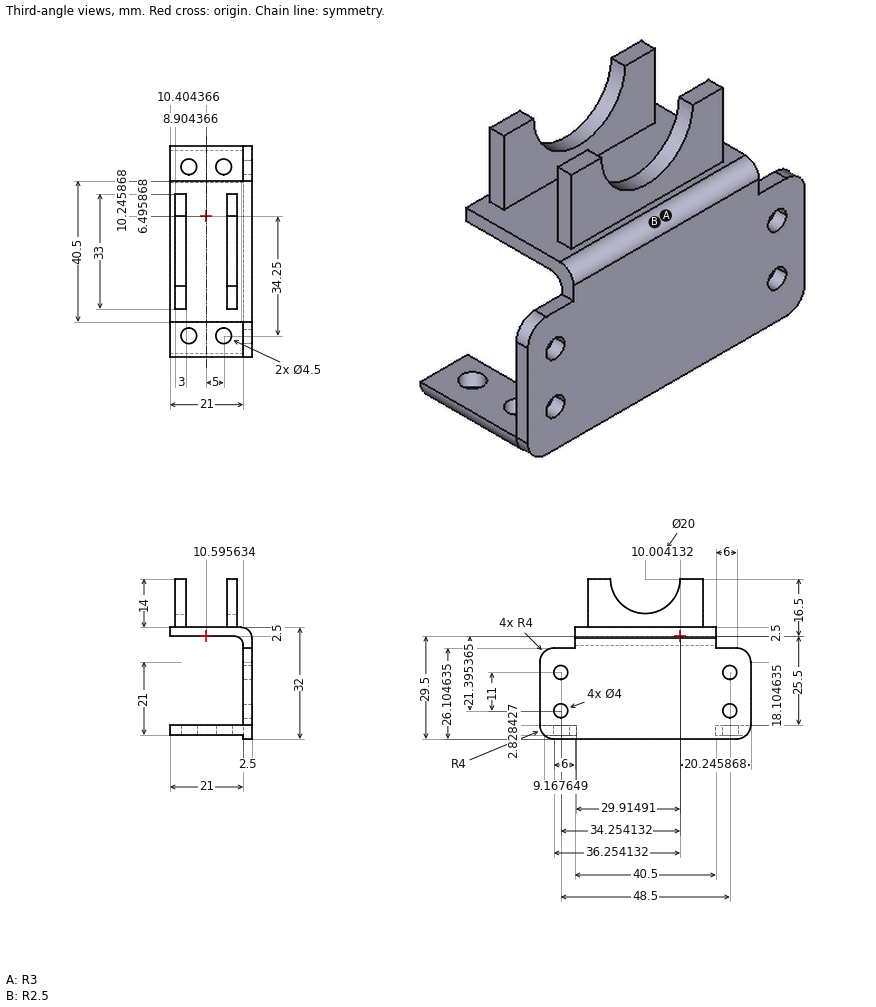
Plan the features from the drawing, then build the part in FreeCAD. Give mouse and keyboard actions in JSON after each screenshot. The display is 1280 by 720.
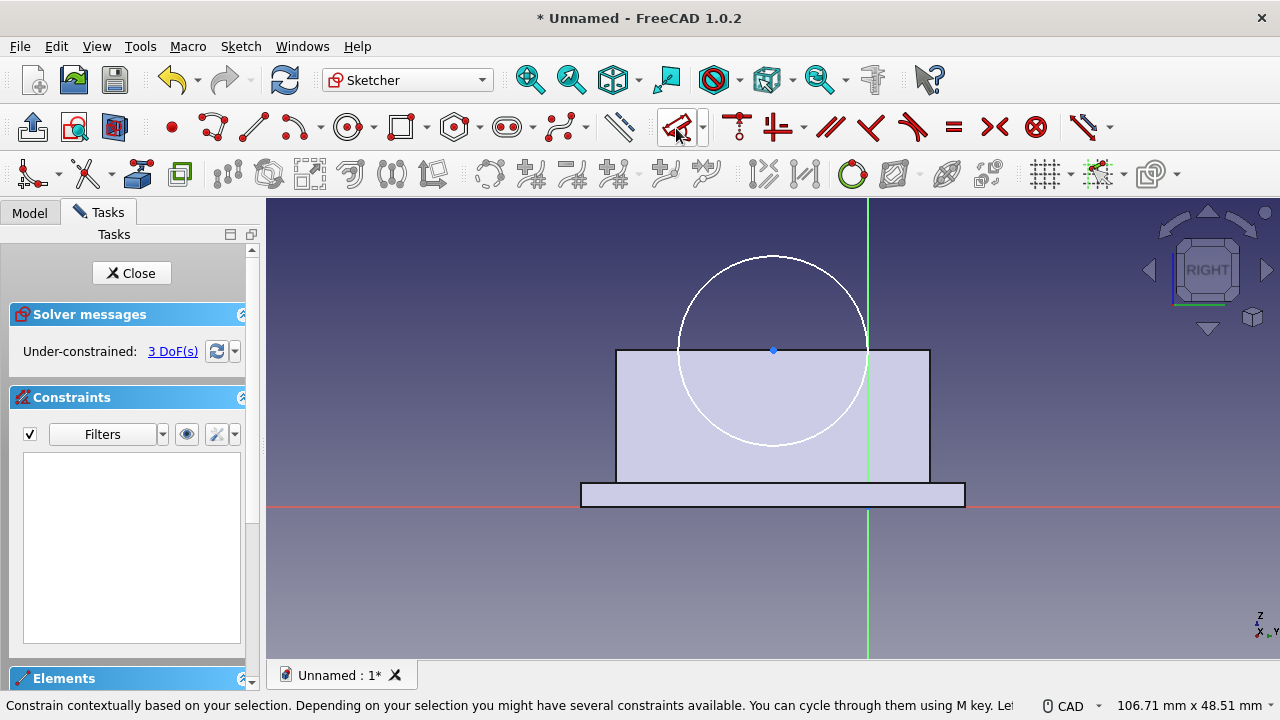
{"action": "left_click", "coordinate": [840, 284]}
{"action": "left_click", "coordinate": [895, 315]}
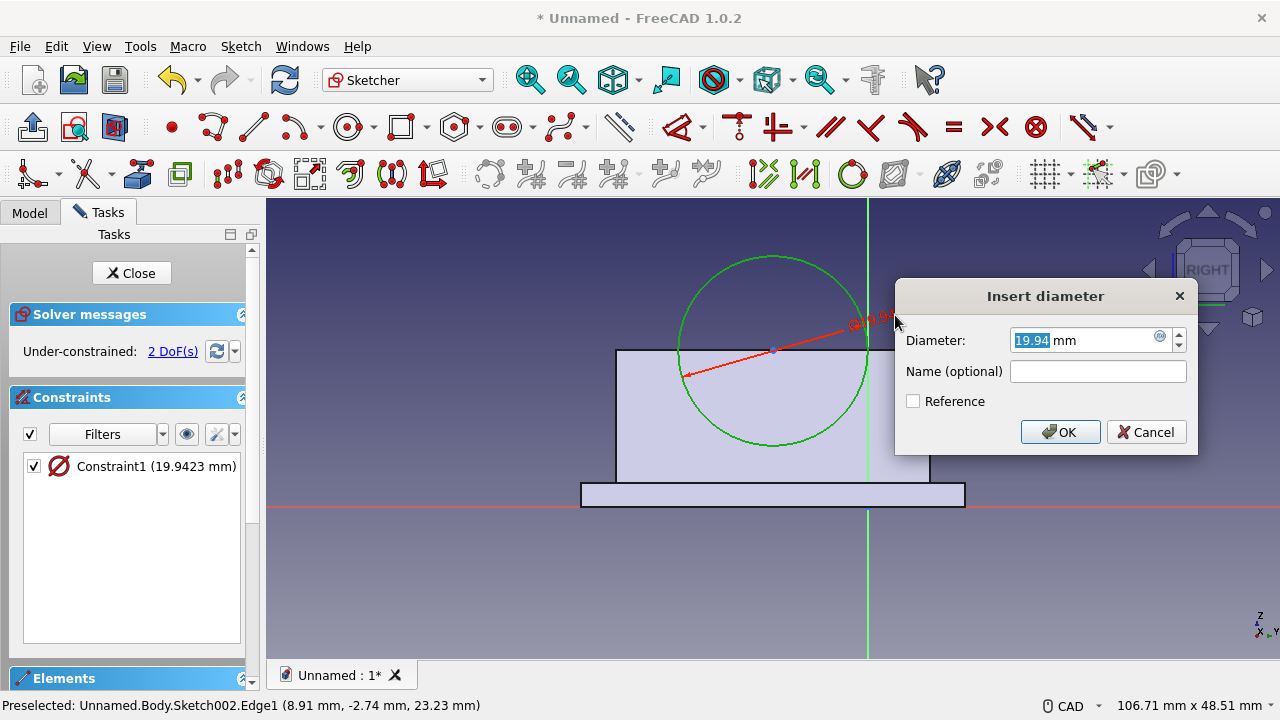
{"action": "type", "text": "20"}
{"action": "key", "text": "Return"}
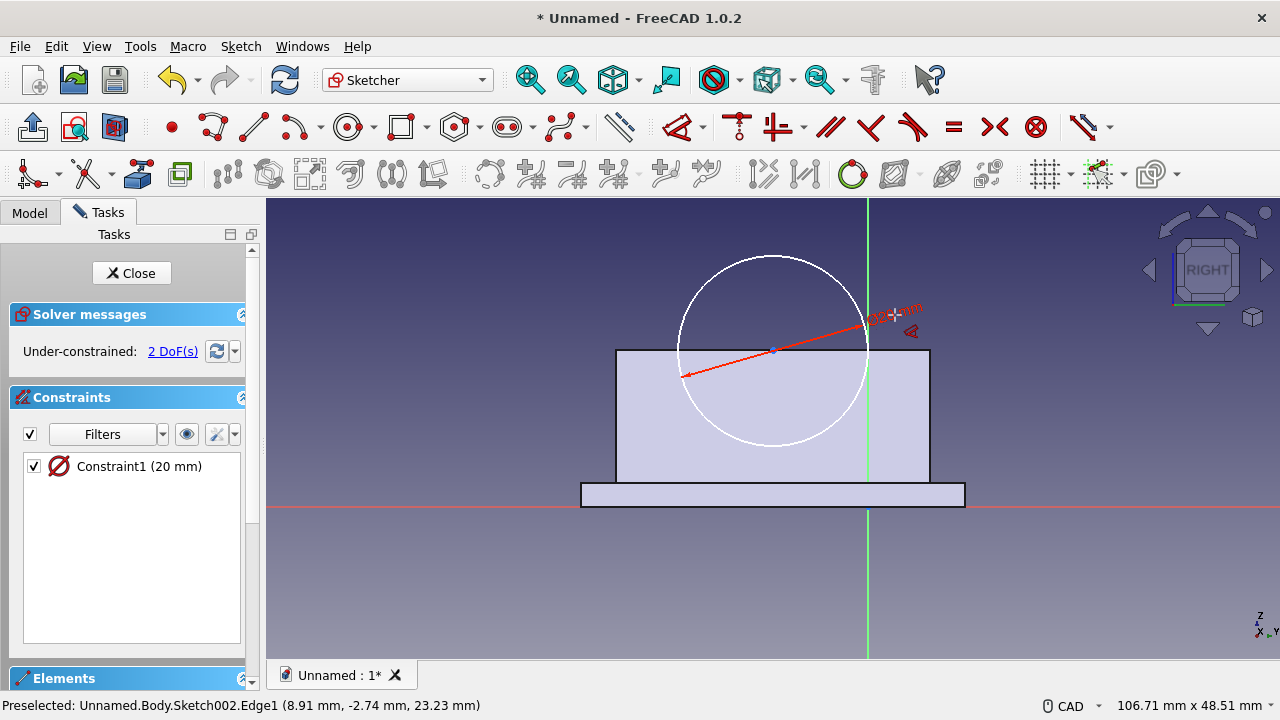
{"action": "left_click", "coordinate": [773, 351]}
{"action": "left_click", "coordinate": [902, 429]}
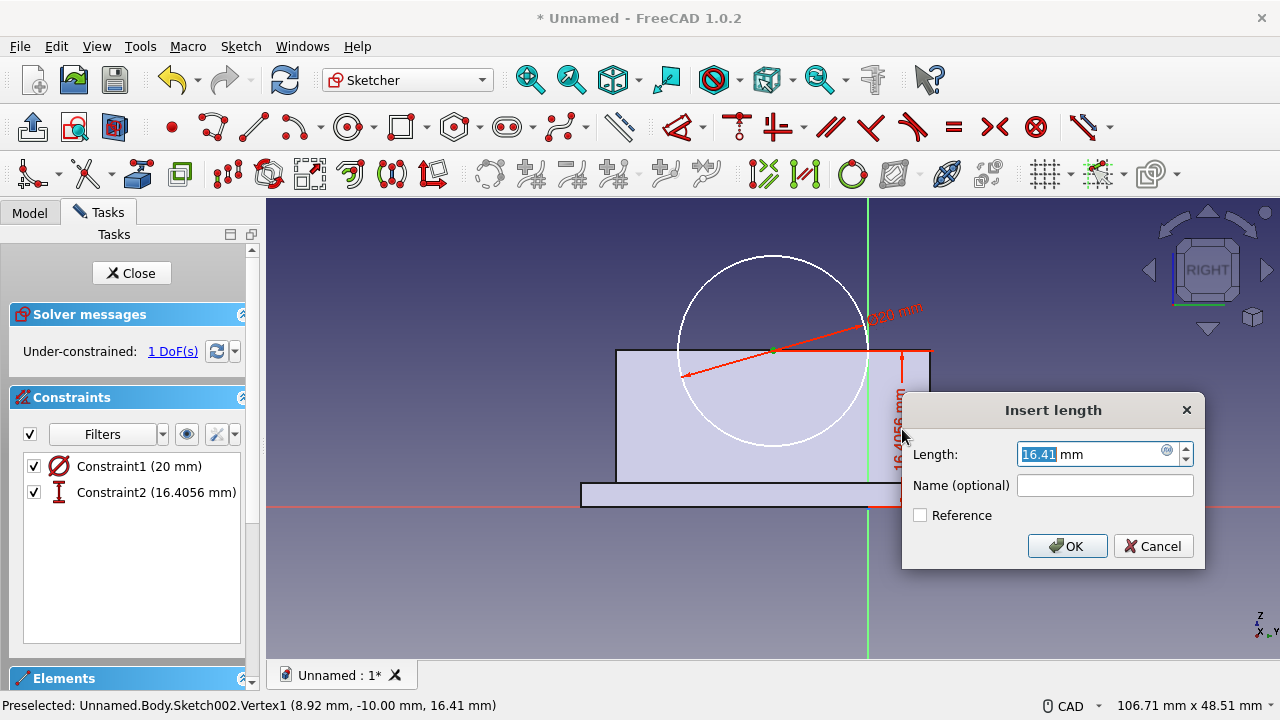
{"action": "type", "text": "16.5"}
{"action": "key", "text": "Return"}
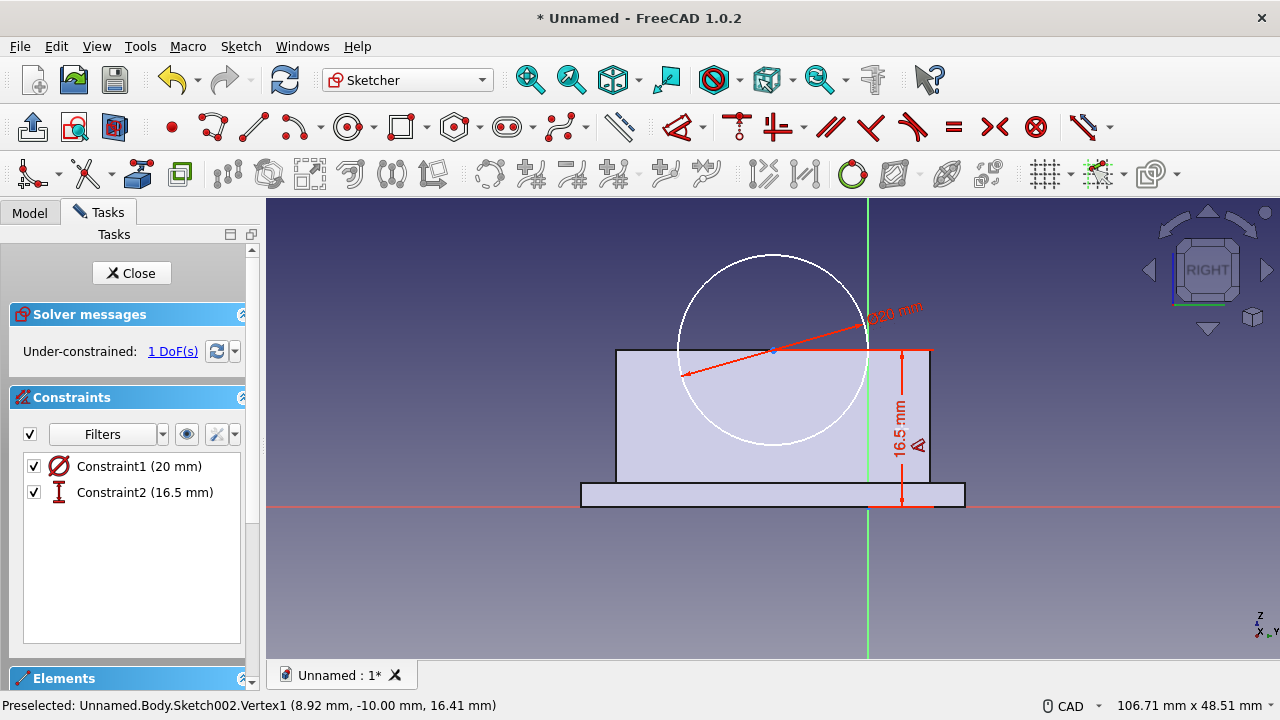
{"action": "left_click", "coordinate": [773, 350]}
{"action": "left_click", "coordinate": [821, 541]}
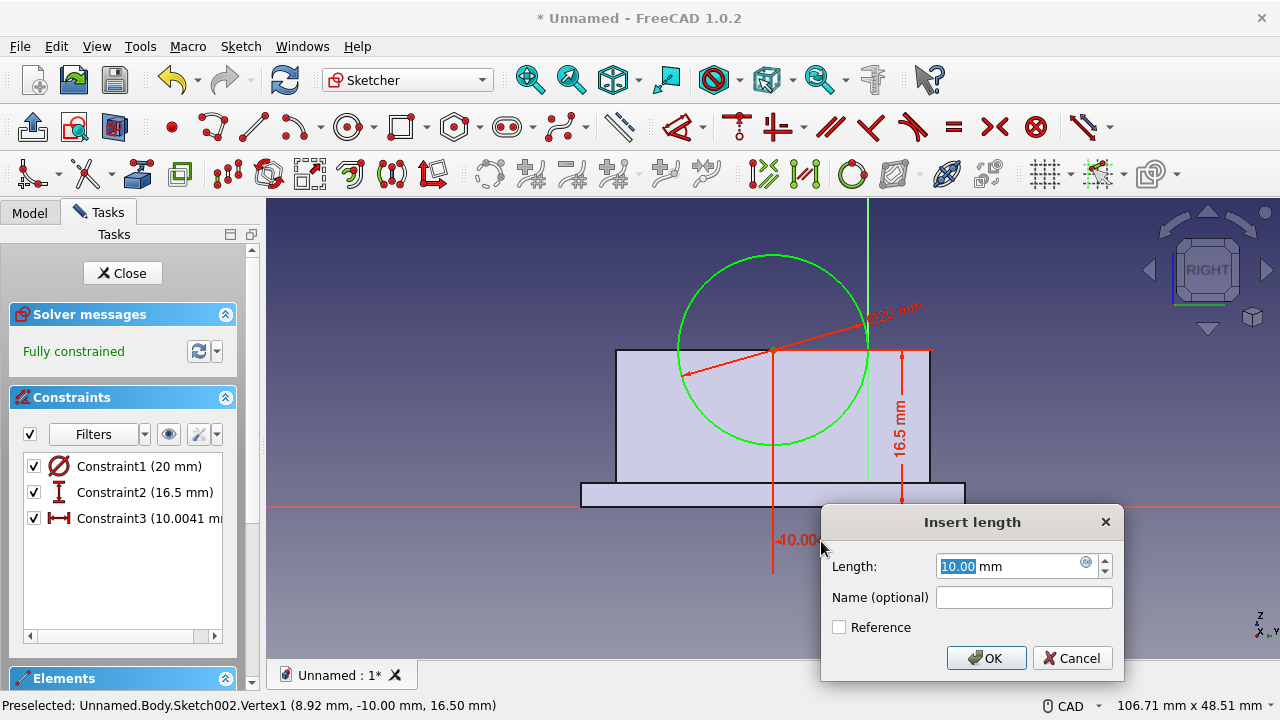
{"action": "type", "text": "10.004132"}
{"action": "key", "text": "Return"}
{"action": "key", "text": "Escape"}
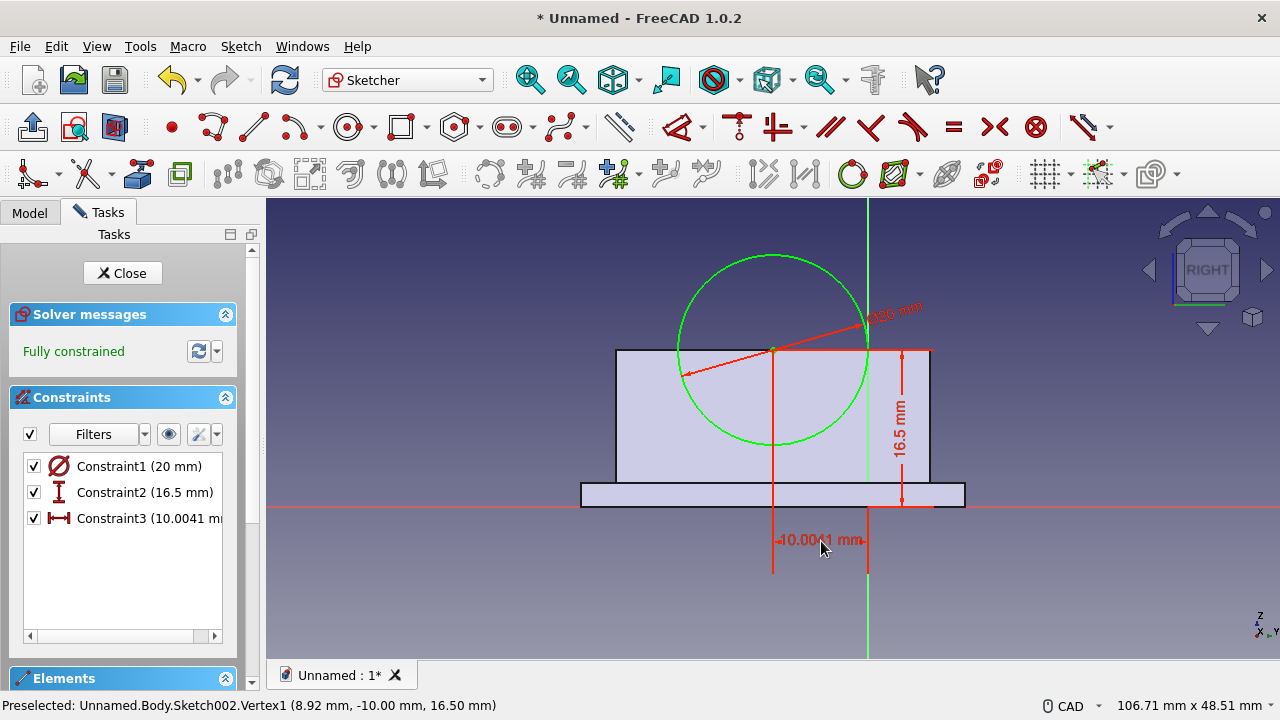
{"action": "left_click", "coordinate": [123, 273]}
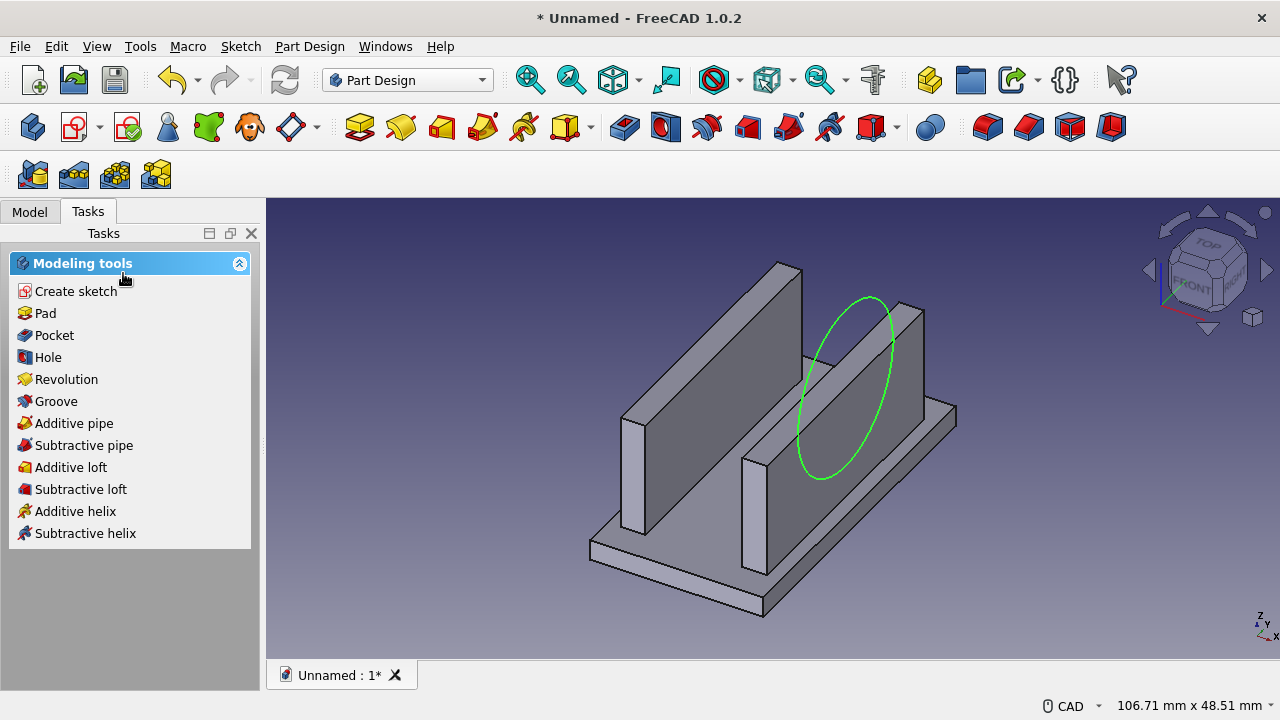
{"action": "left_click", "coordinate": [625, 128]}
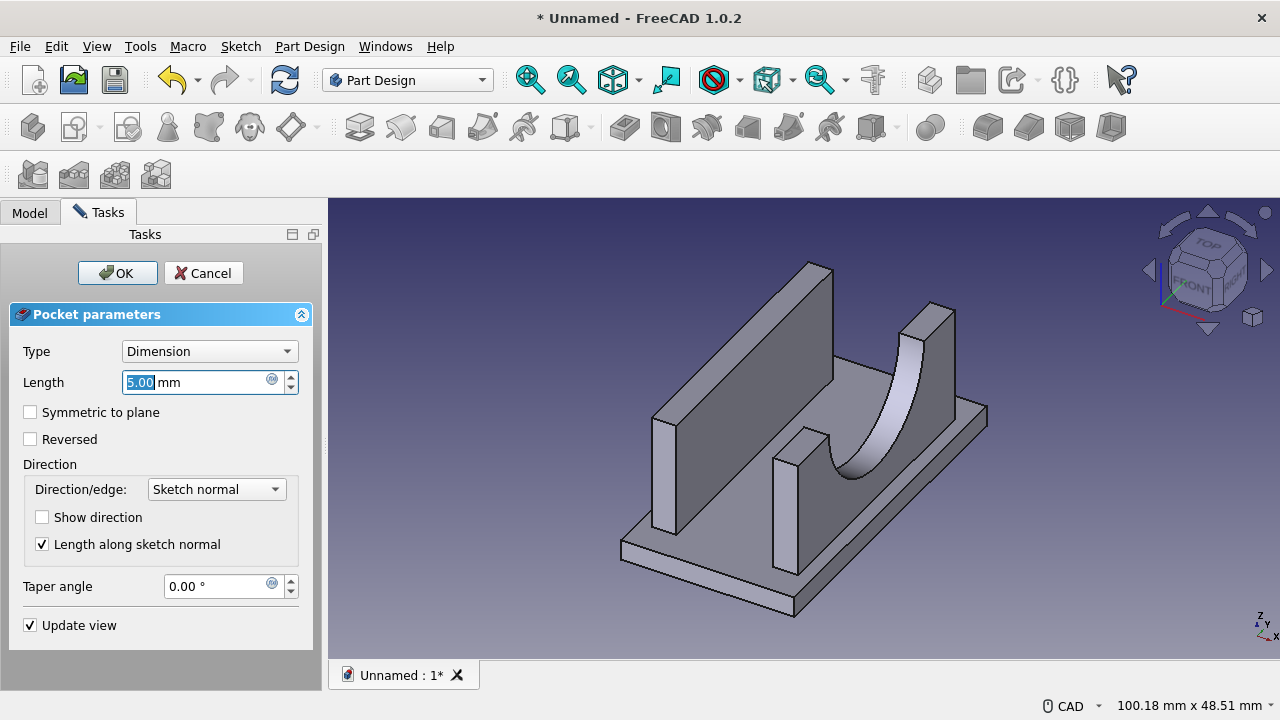
{"action": "left_click", "coordinate": [210, 352]}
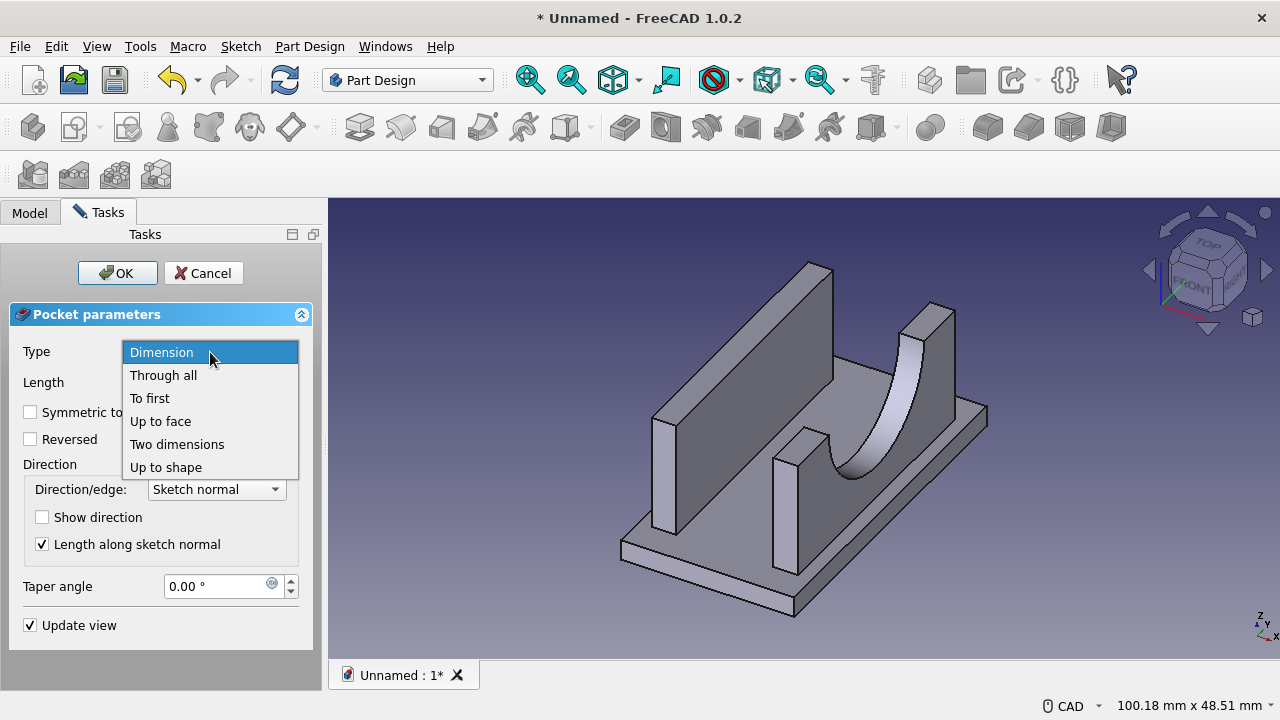
{"action": "left_click", "coordinate": [208, 376]}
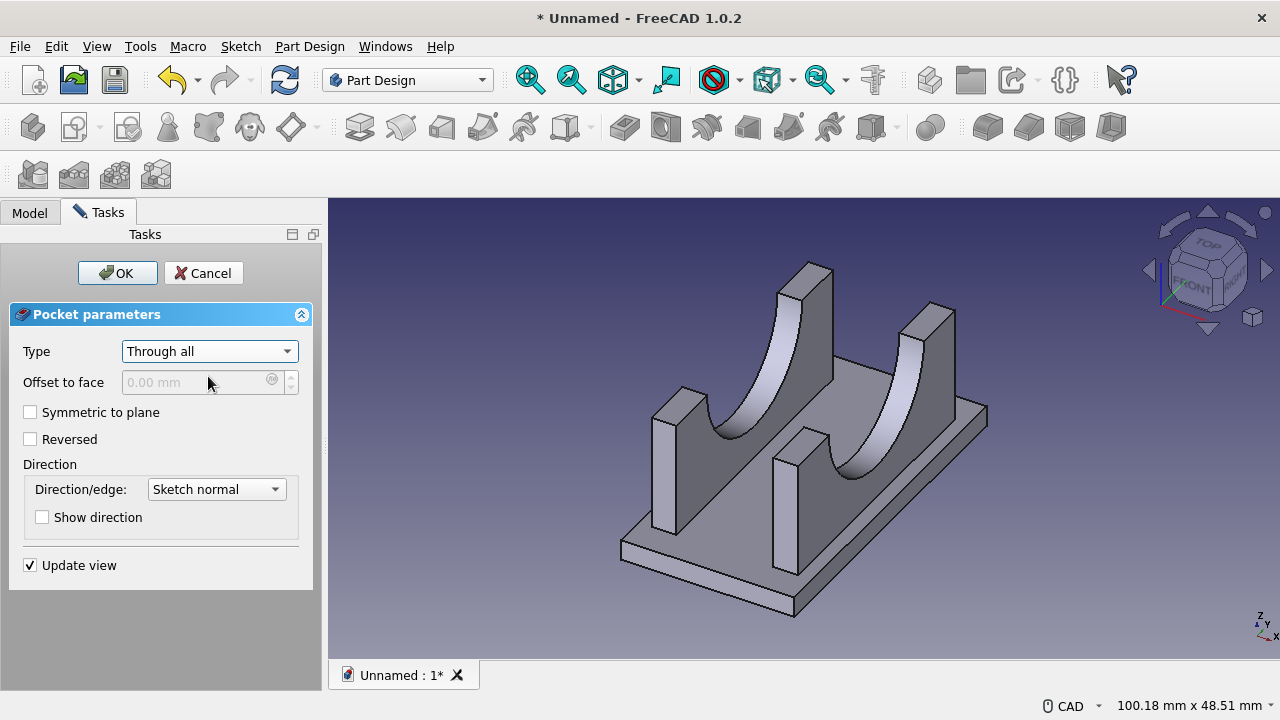
{"action": "left_click", "coordinate": [118, 273]}